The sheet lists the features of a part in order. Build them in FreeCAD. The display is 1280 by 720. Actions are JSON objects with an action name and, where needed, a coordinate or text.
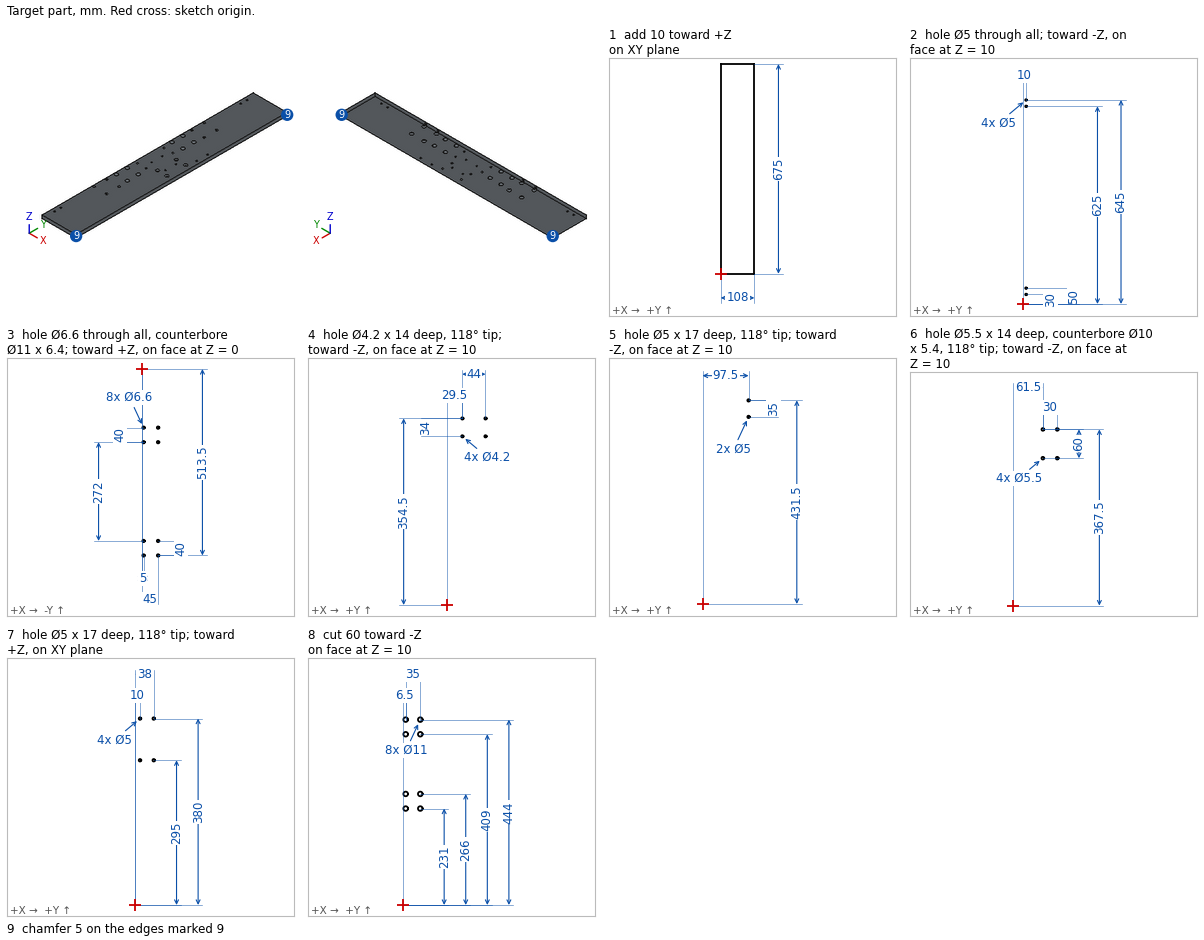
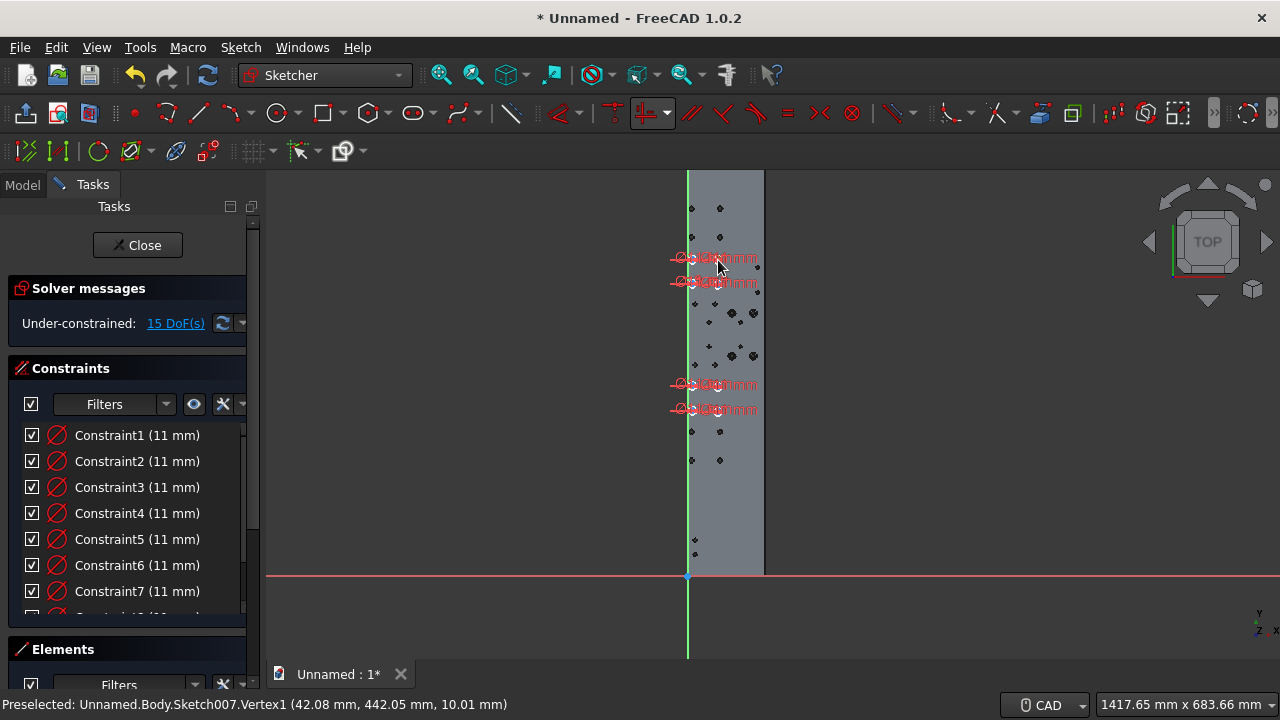
{"action": "left_click", "coordinate": [718, 285]}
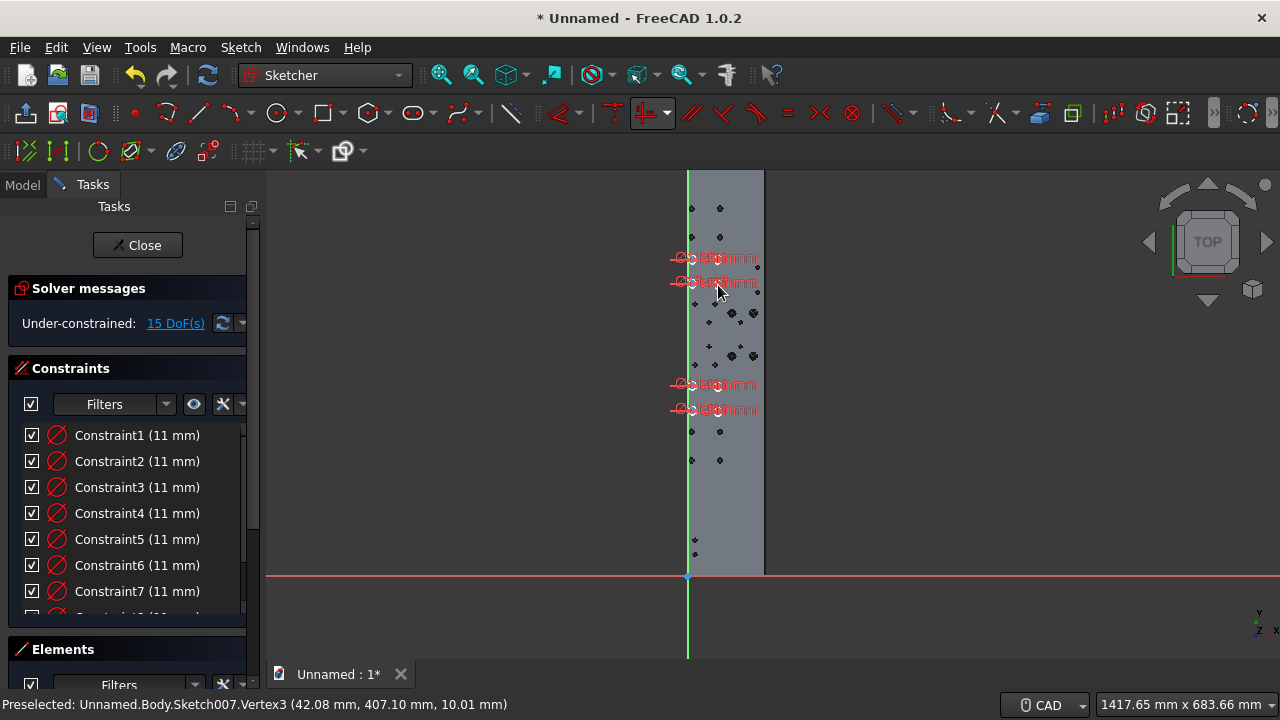
{"action": "left_click", "coordinate": [670, 114]}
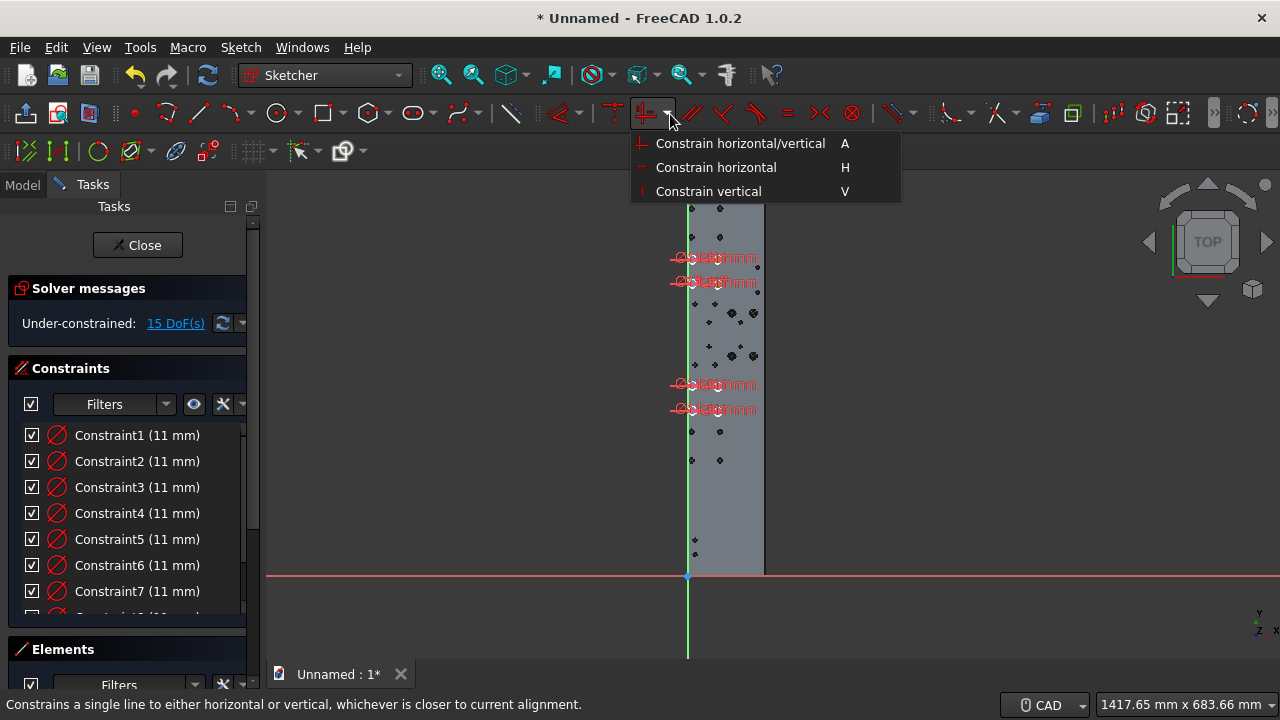
{"action": "left_click", "coordinate": [766, 191]}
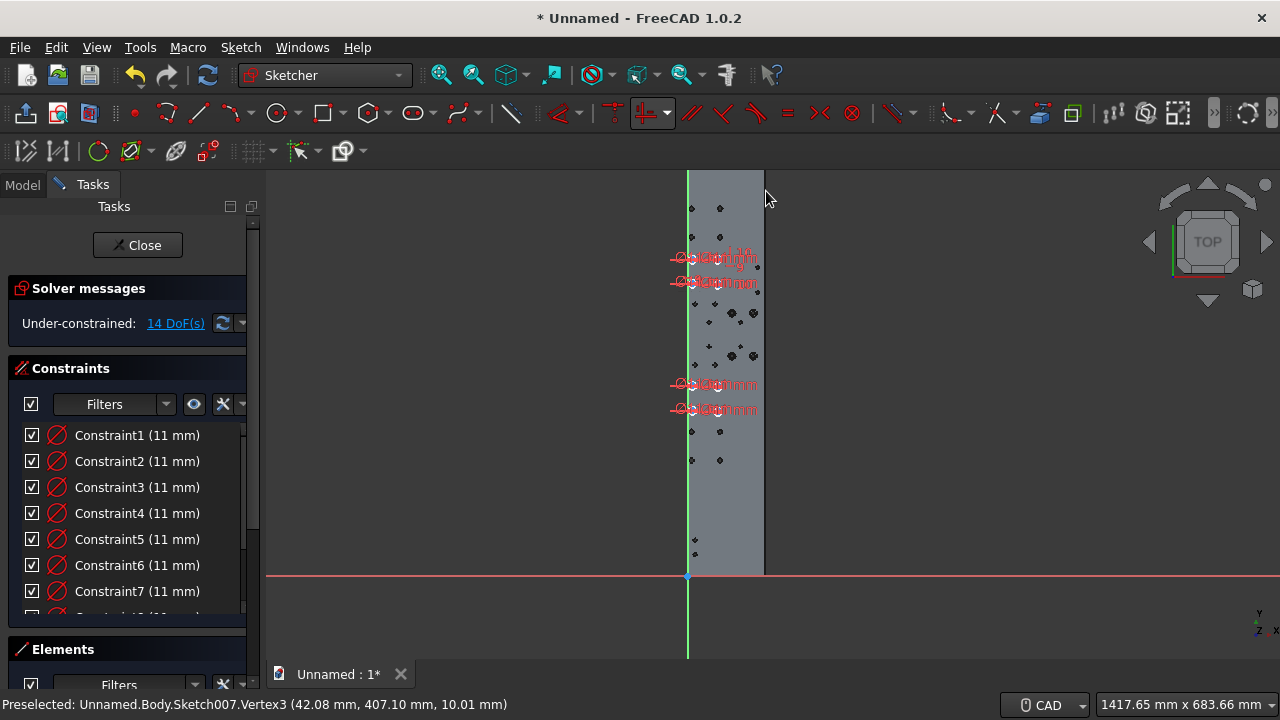
{"action": "left_click", "coordinate": [693, 260]}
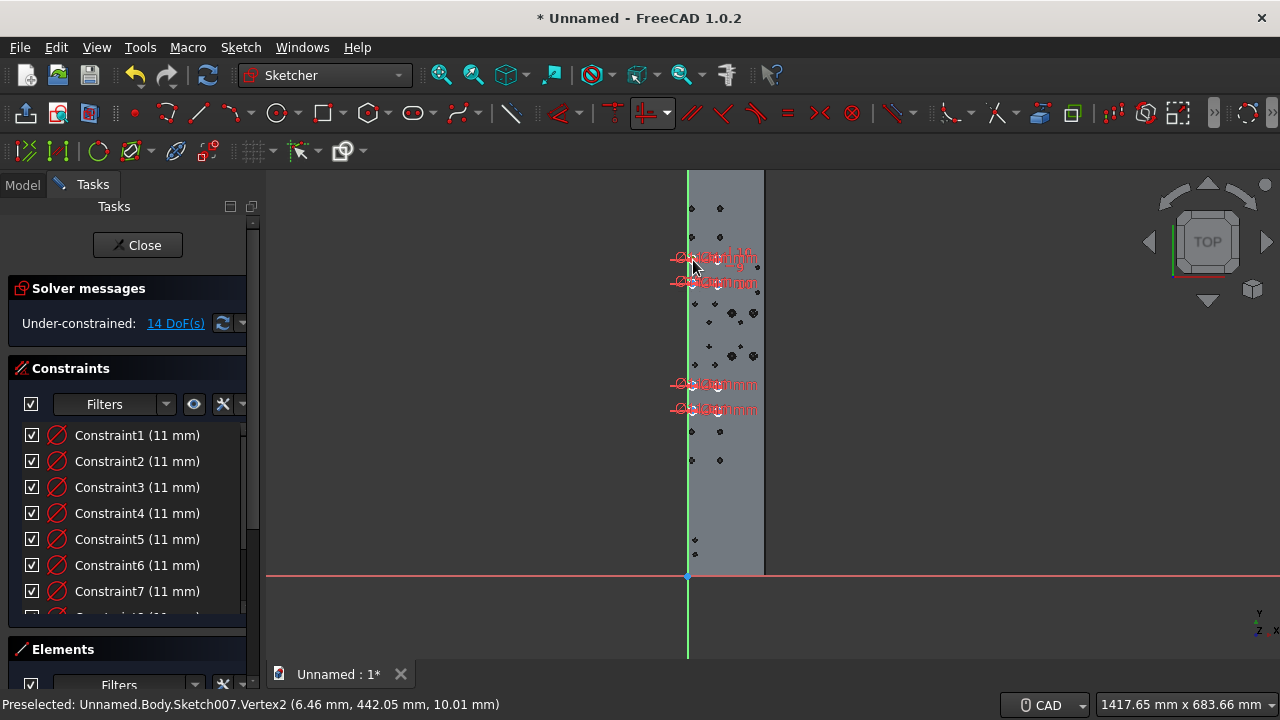
{"action": "left_click", "coordinate": [691, 286]}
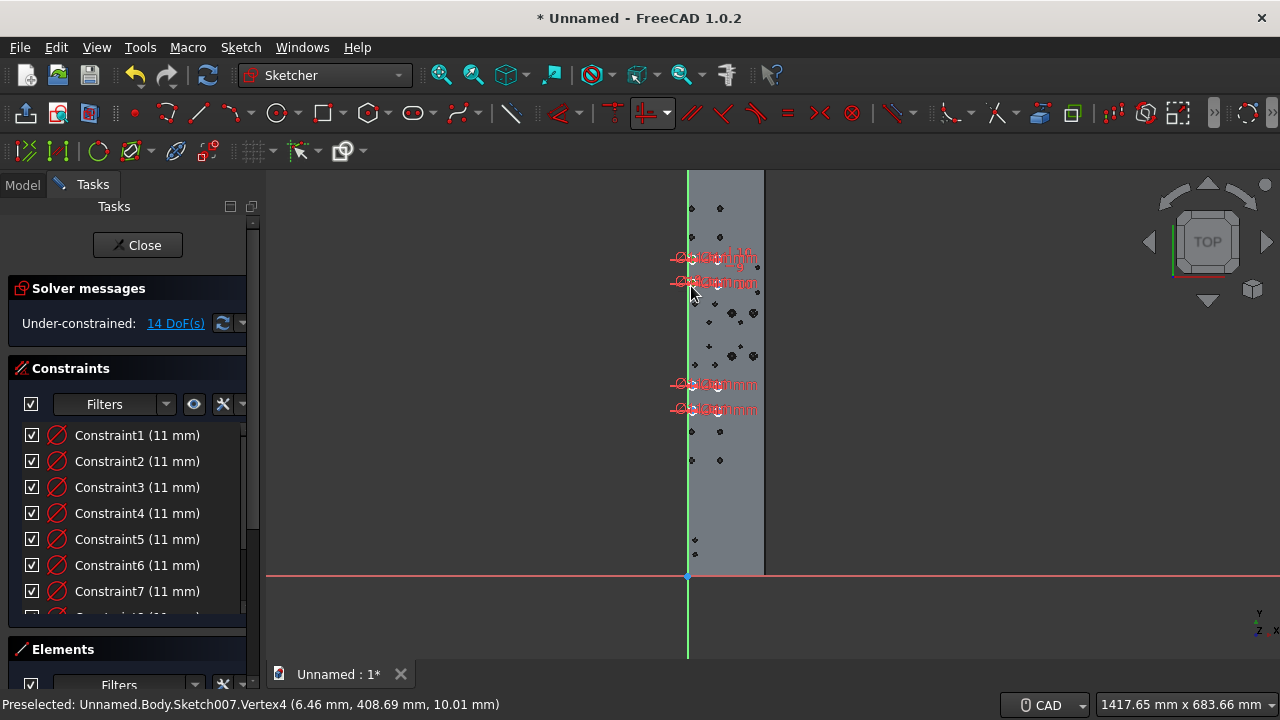
{"action": "key", "text": "v"}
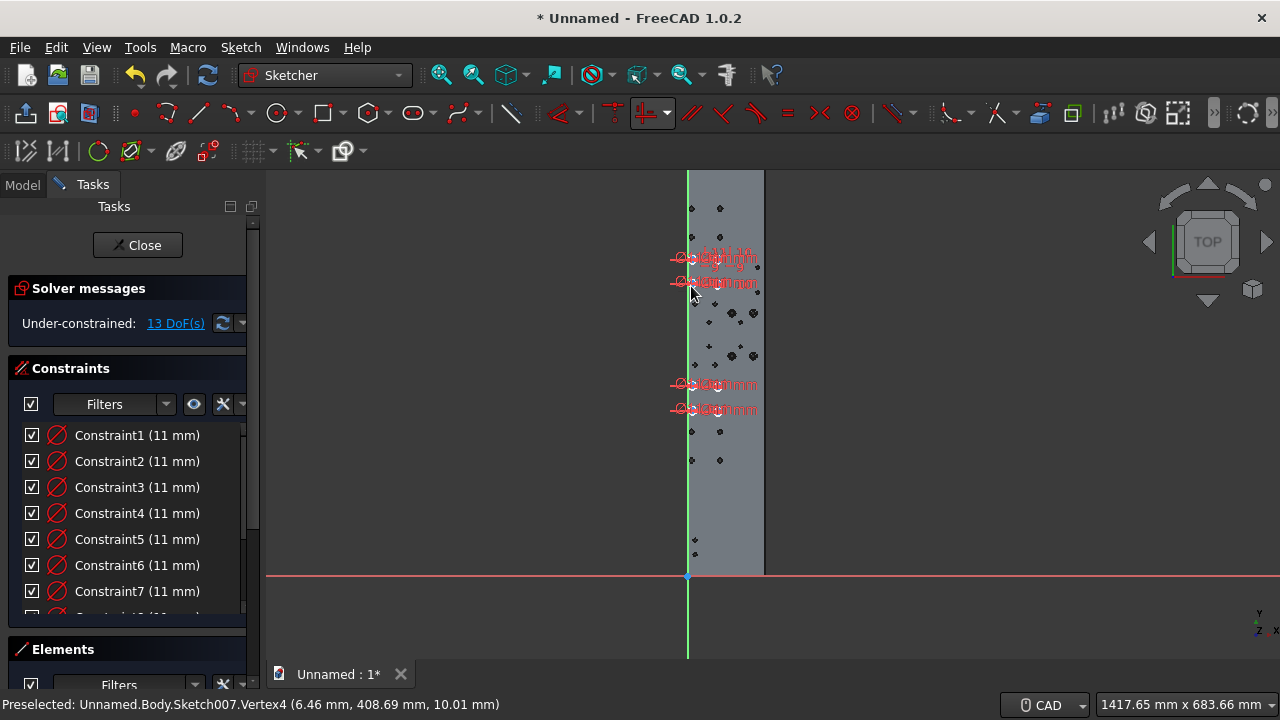
{"action": "scroll", "coordinate": [718, 285], "scroll_direction": "up", "scroll_amount": 4}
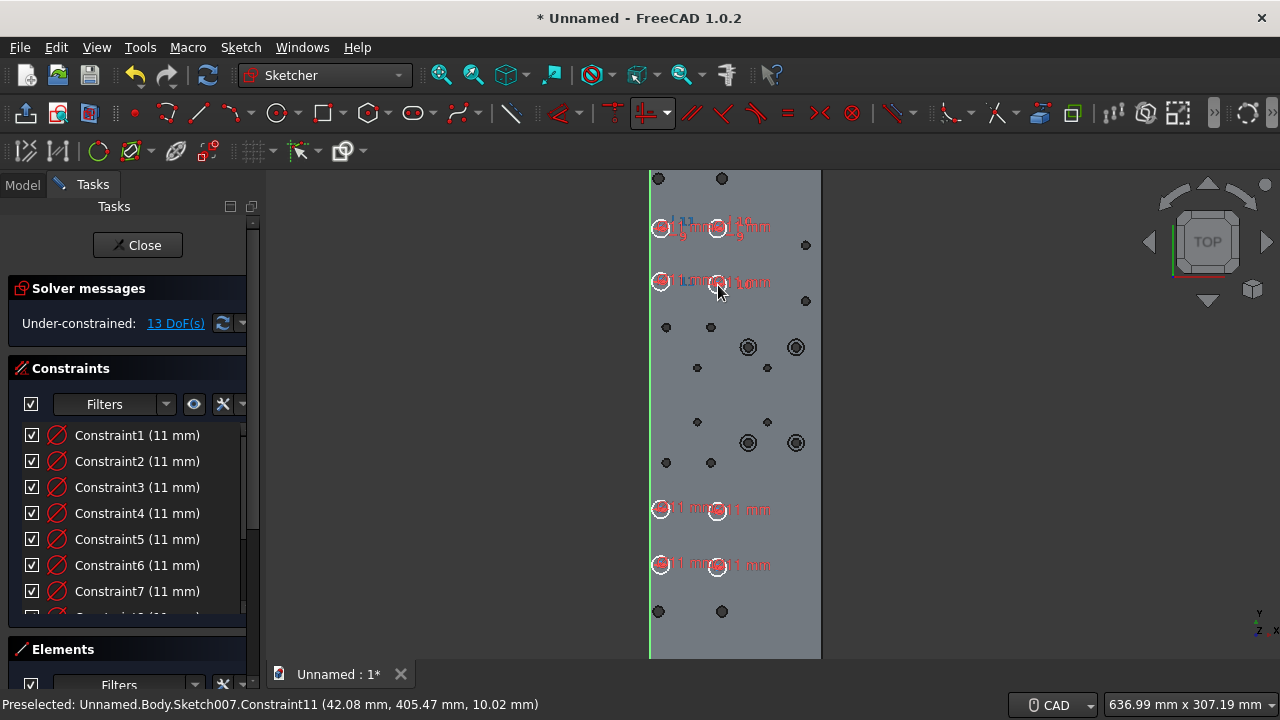
{"action": "left_click", "coordinate": [717, 284]}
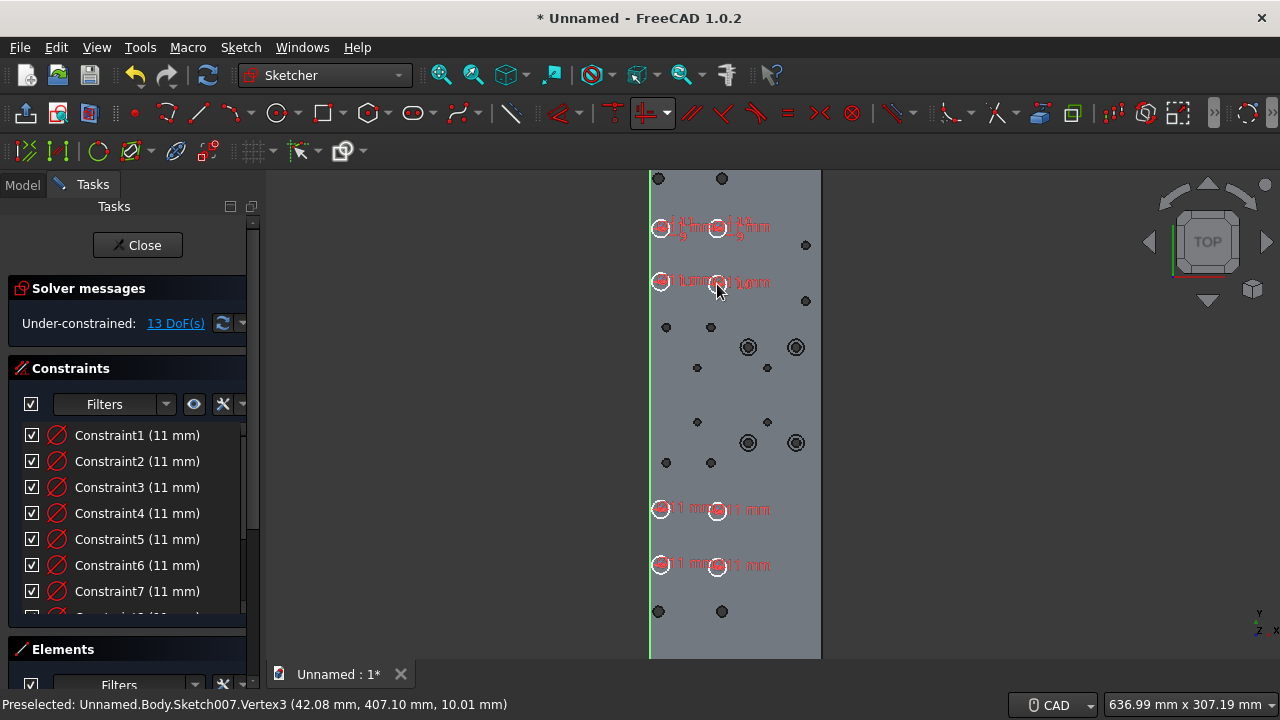
{"action": "left_click", "coordinate": [661, 282]}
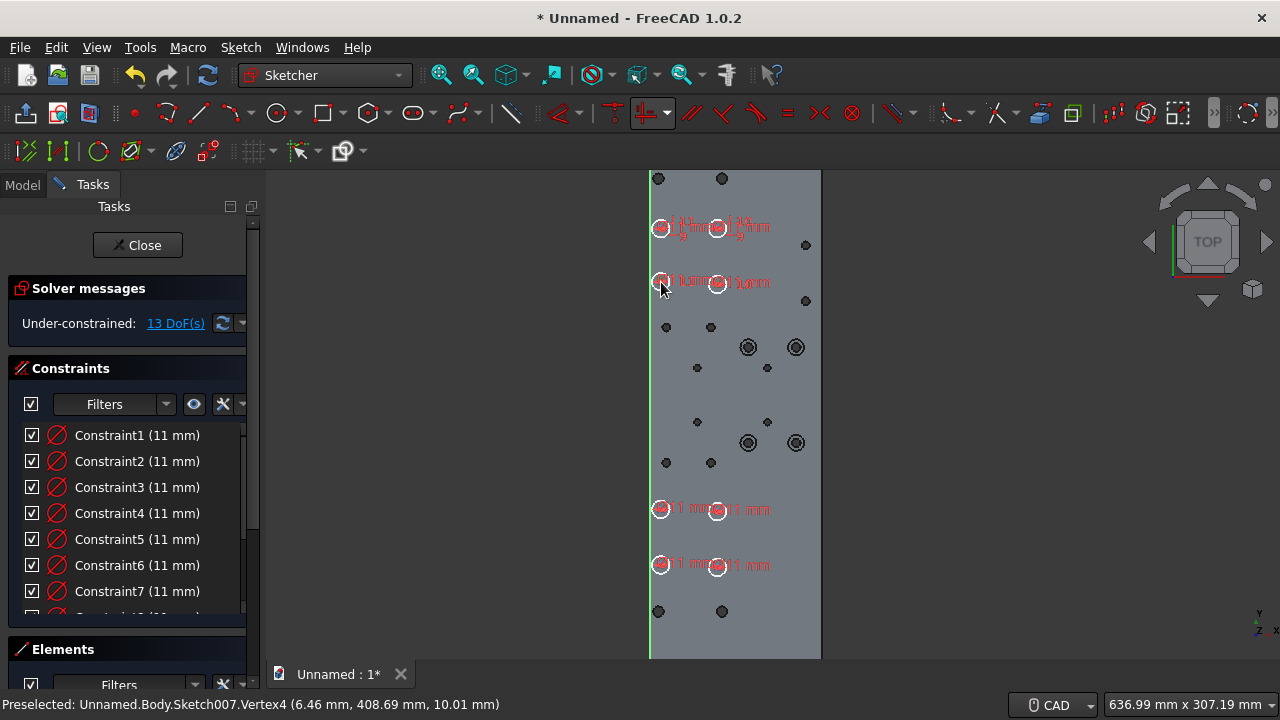
{"action": "key", "text": "h"}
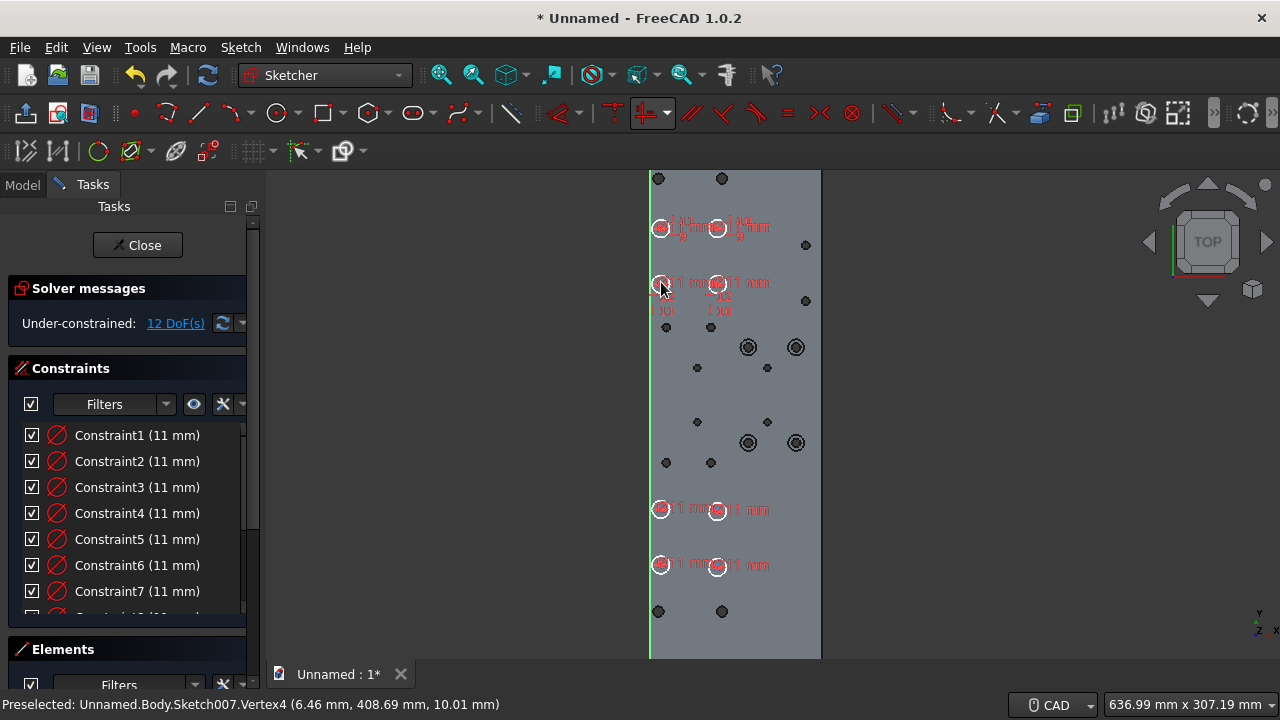
{"action": "left_click", "coordinate": [717, 284]}